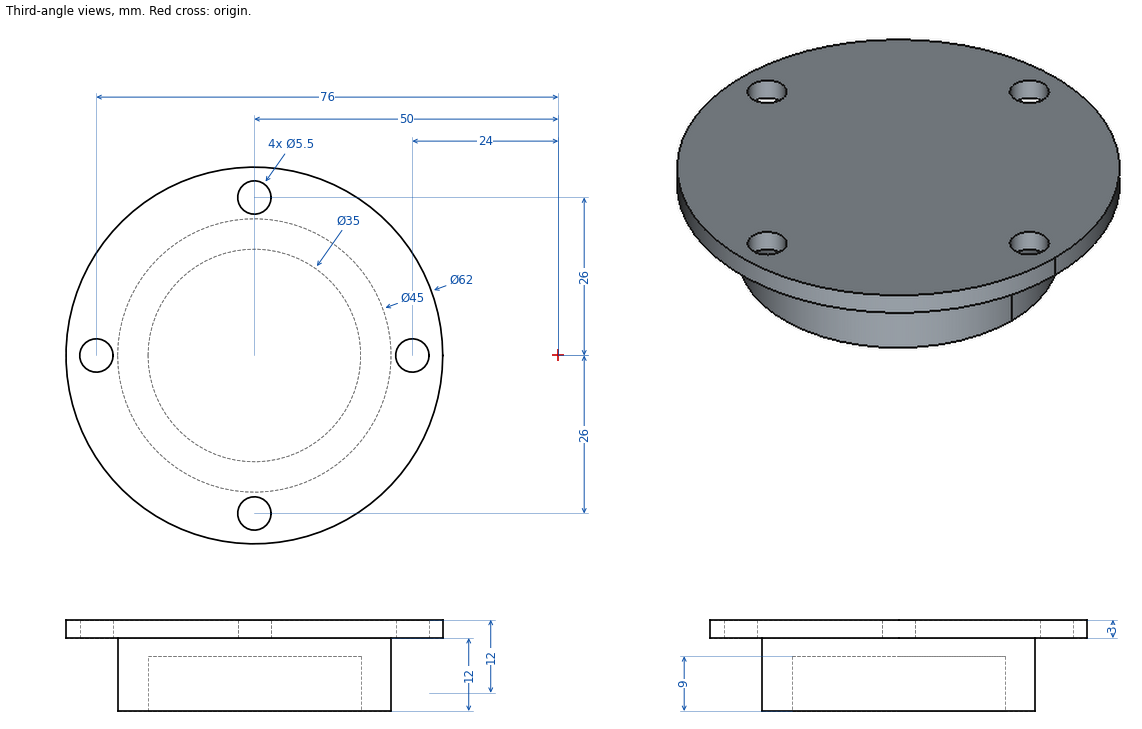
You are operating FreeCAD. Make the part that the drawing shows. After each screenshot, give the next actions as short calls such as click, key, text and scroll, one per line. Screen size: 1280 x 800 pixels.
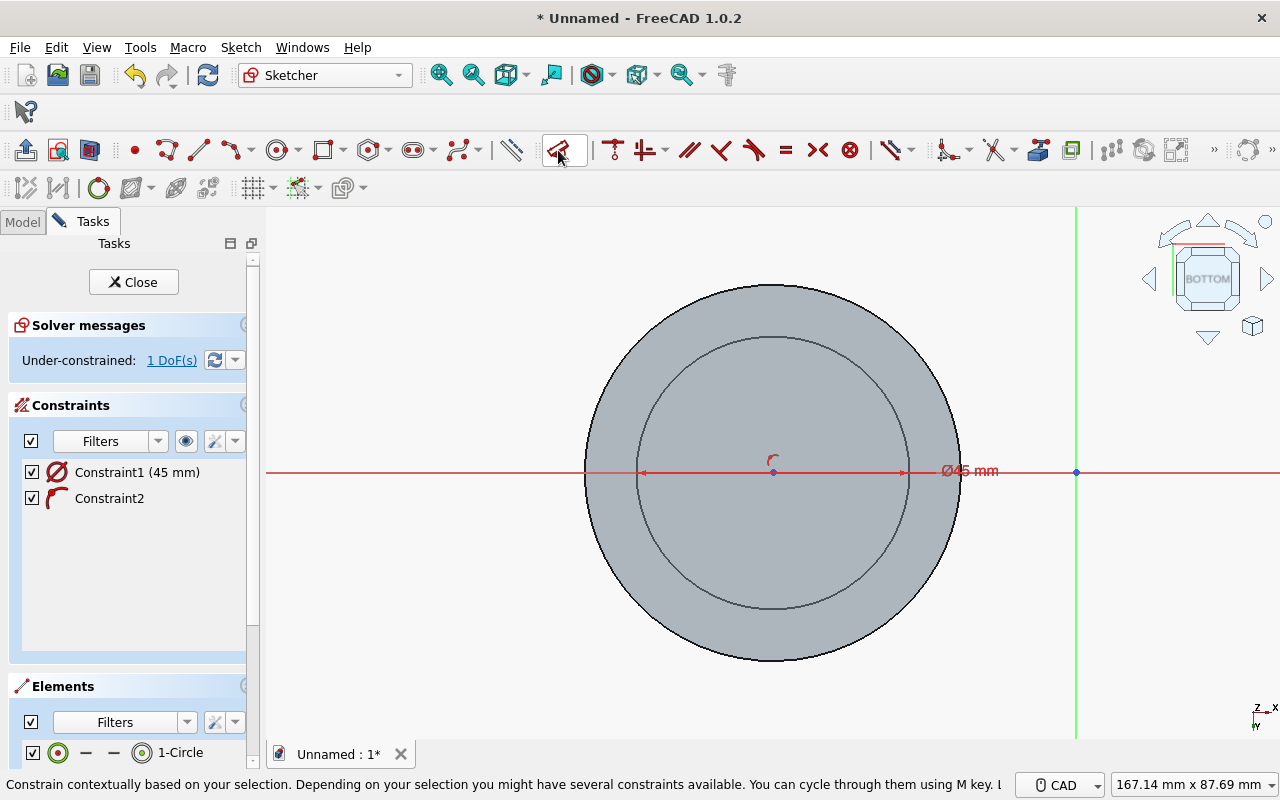
click(773, 473)
click(925, 507)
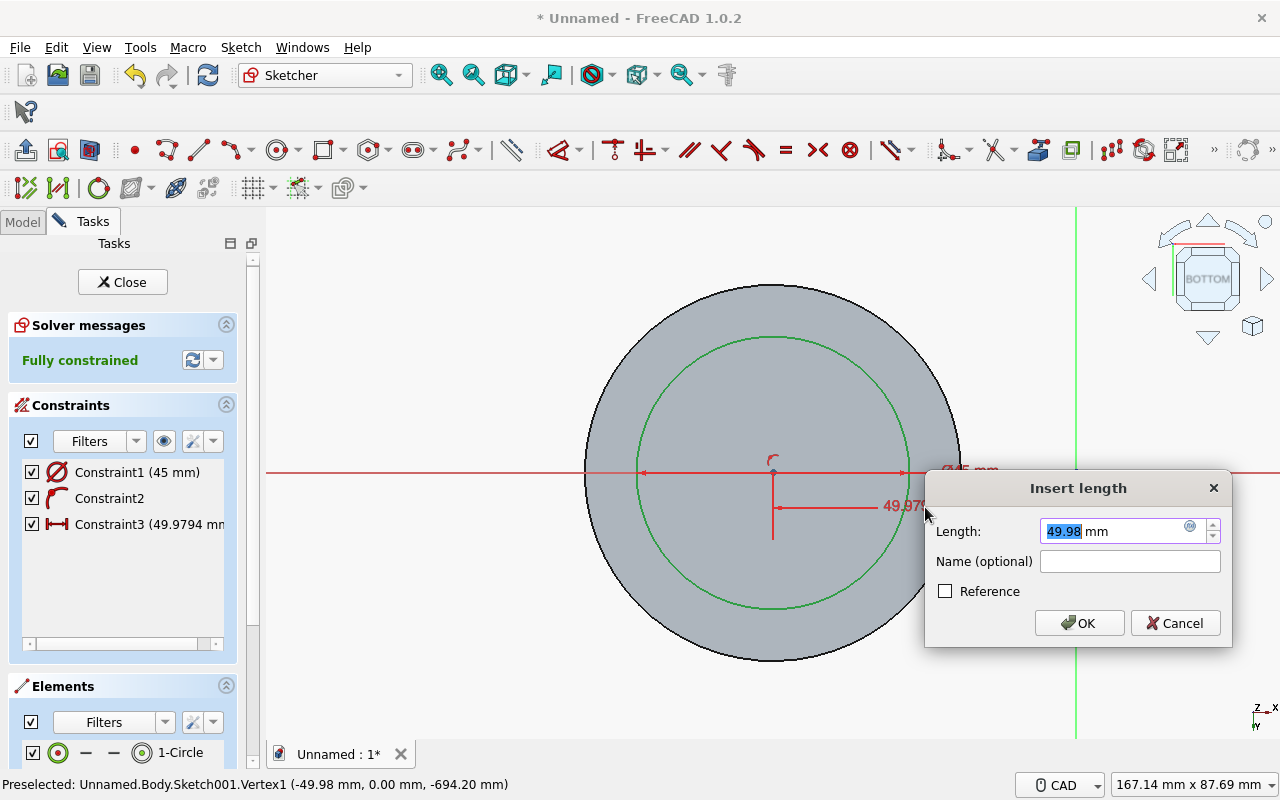
text(50)
key(Return)
key(Escape)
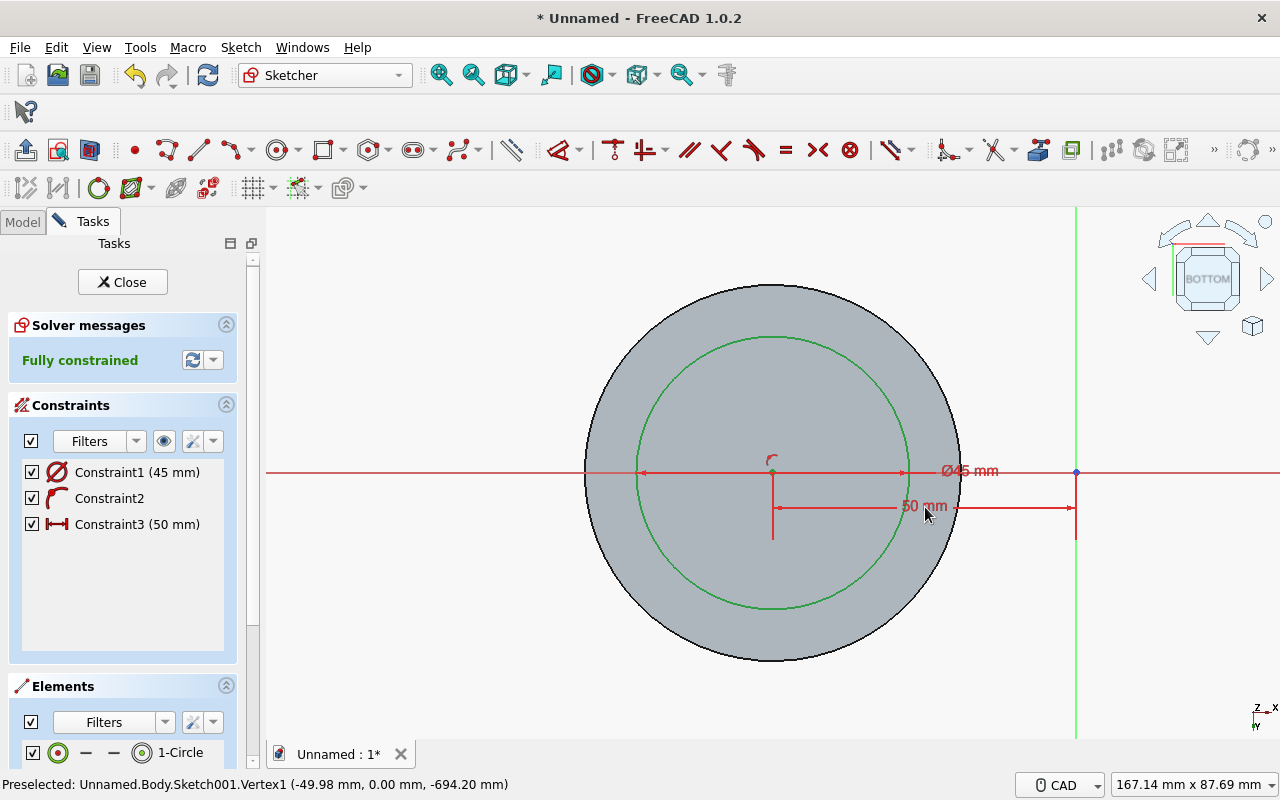
click(123, 282)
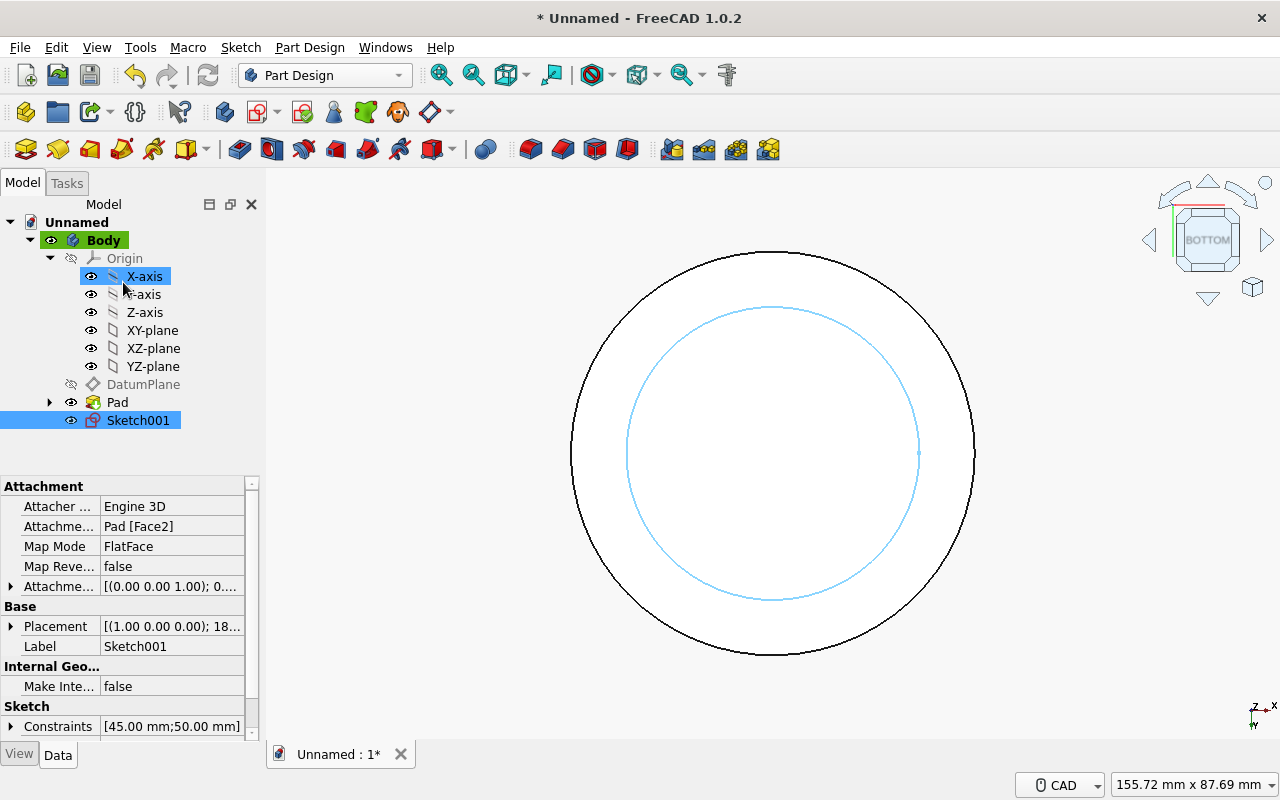
click(26, 150)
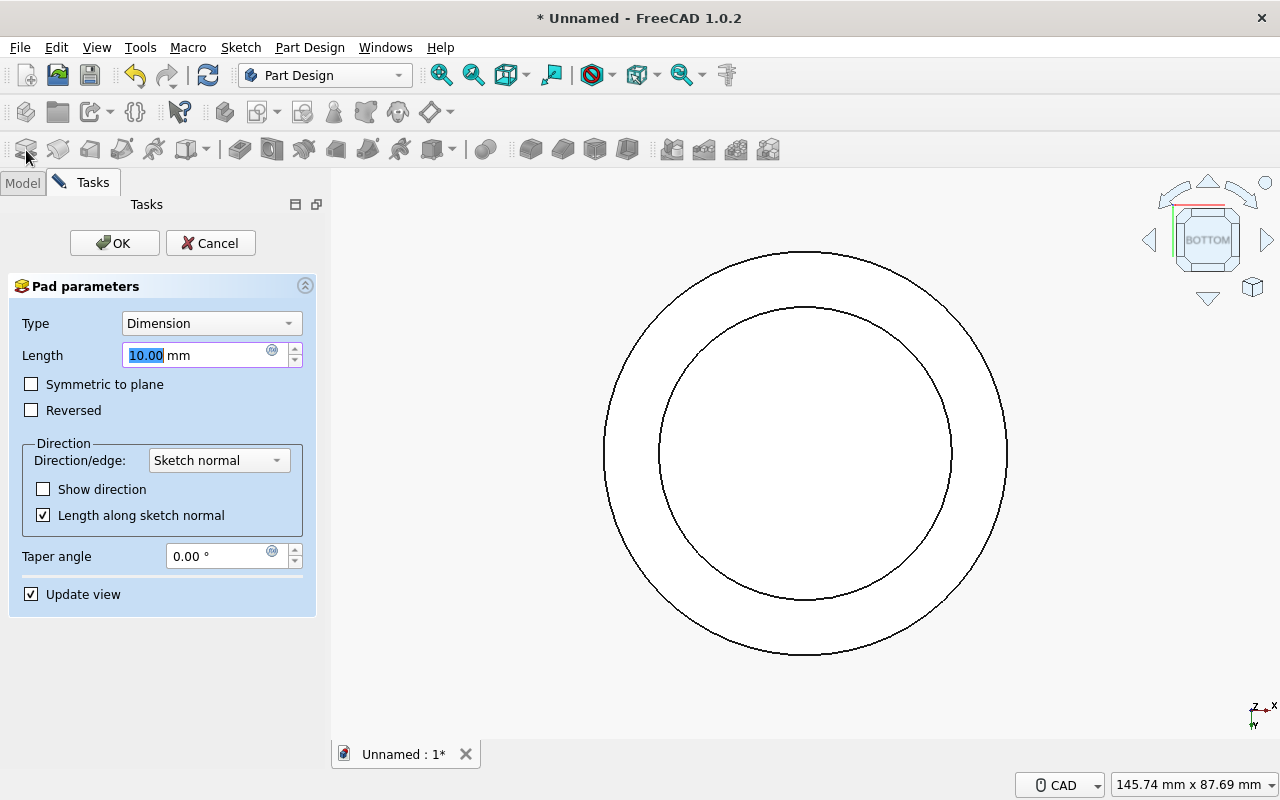
text(12)
key(Tab)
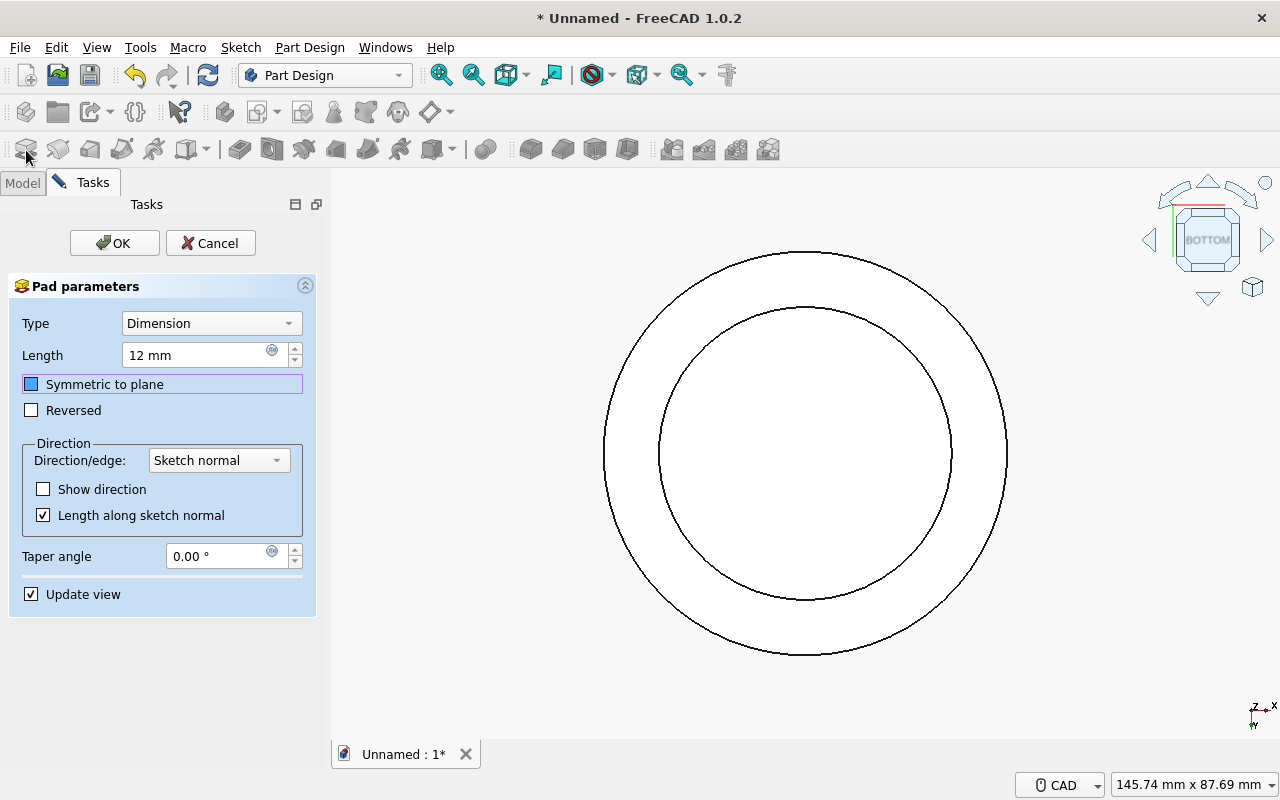
click(115, 243)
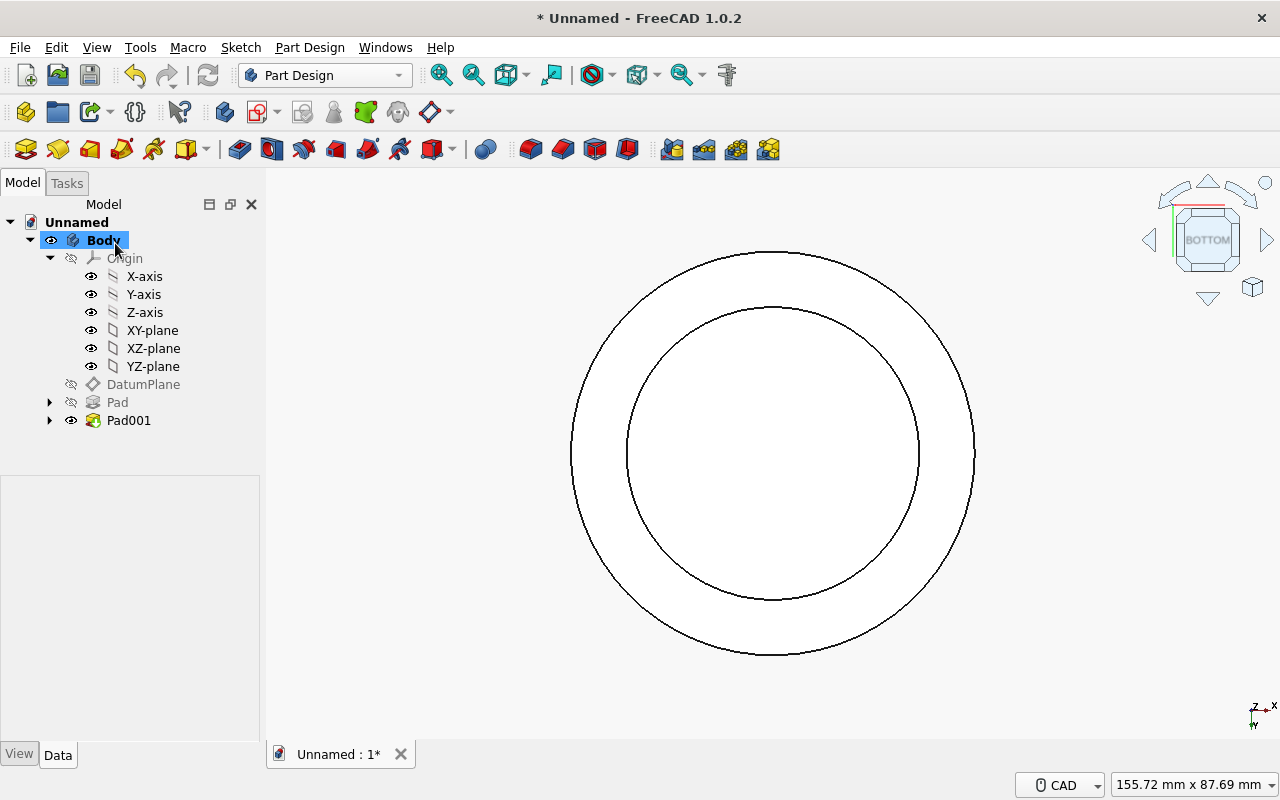
click(773, 453)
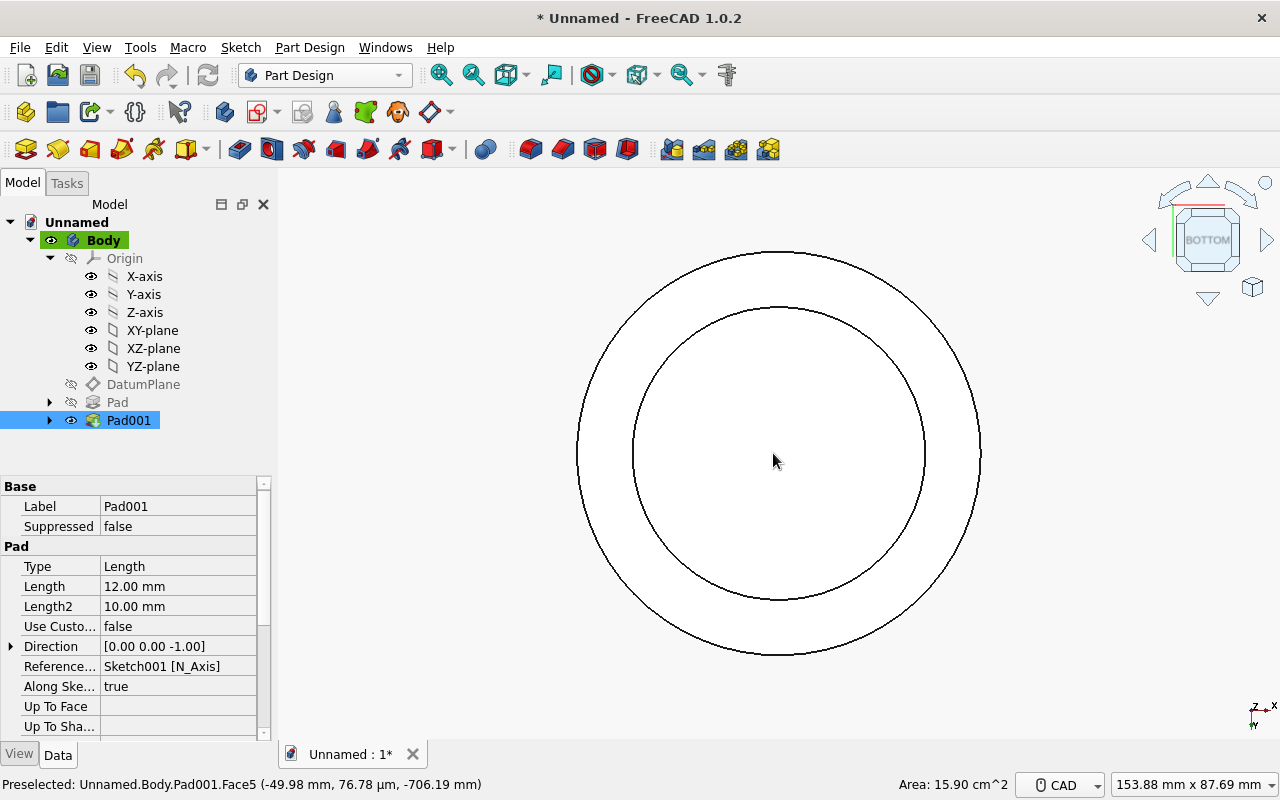
click(258, 112)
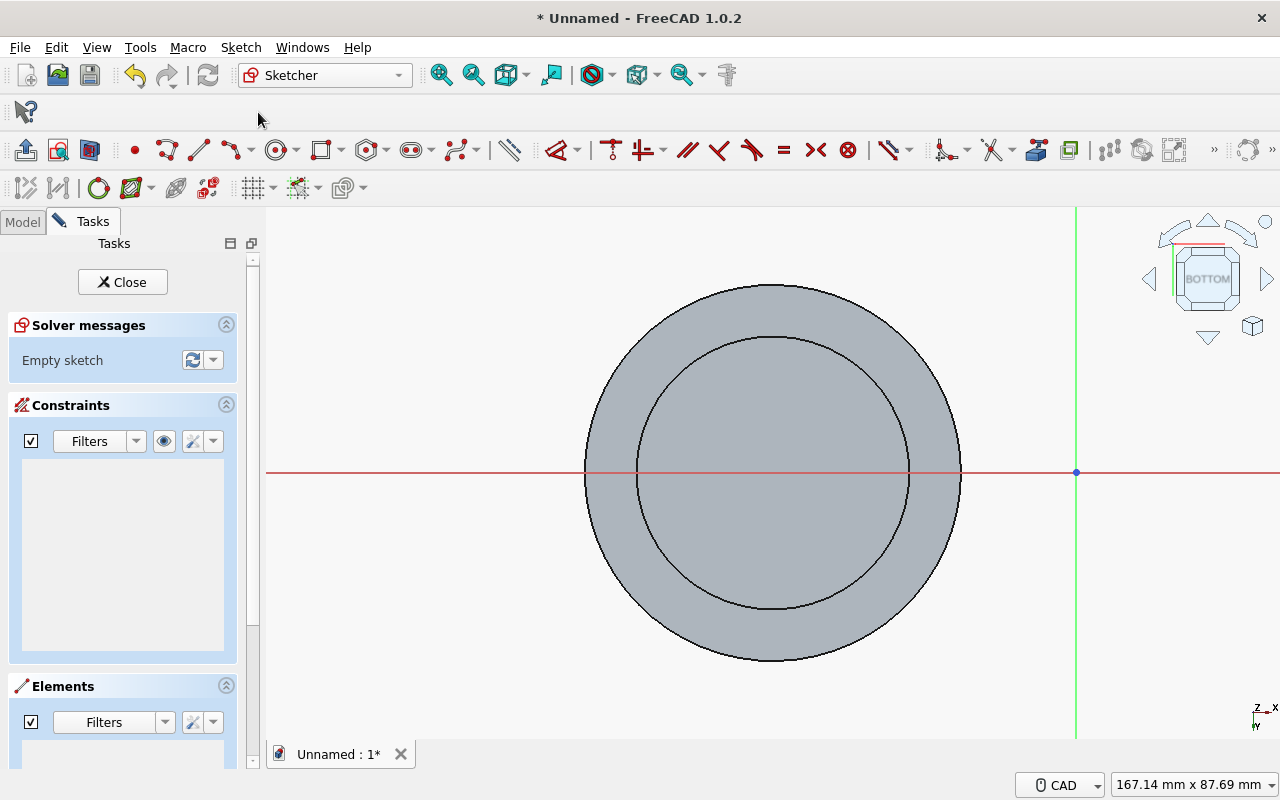
scroll(1115, 473, up, 2)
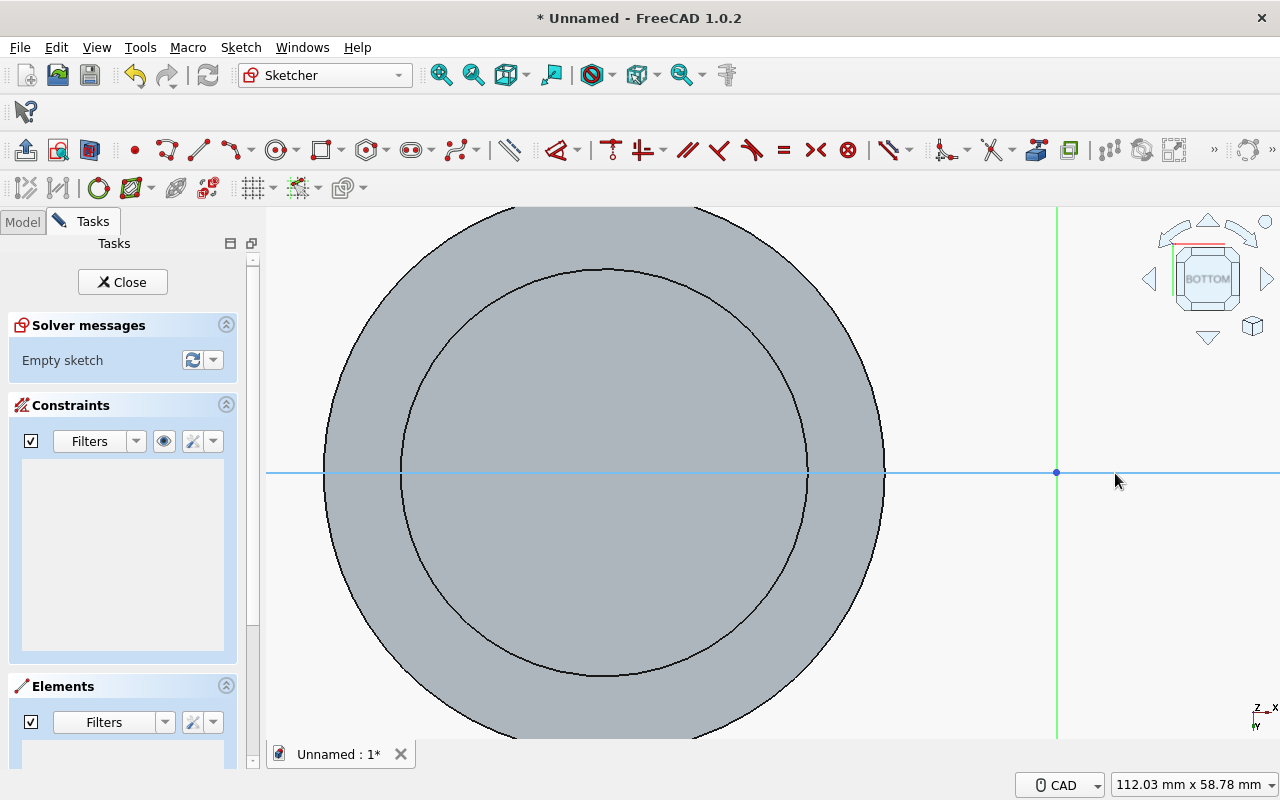
click(276, 150)